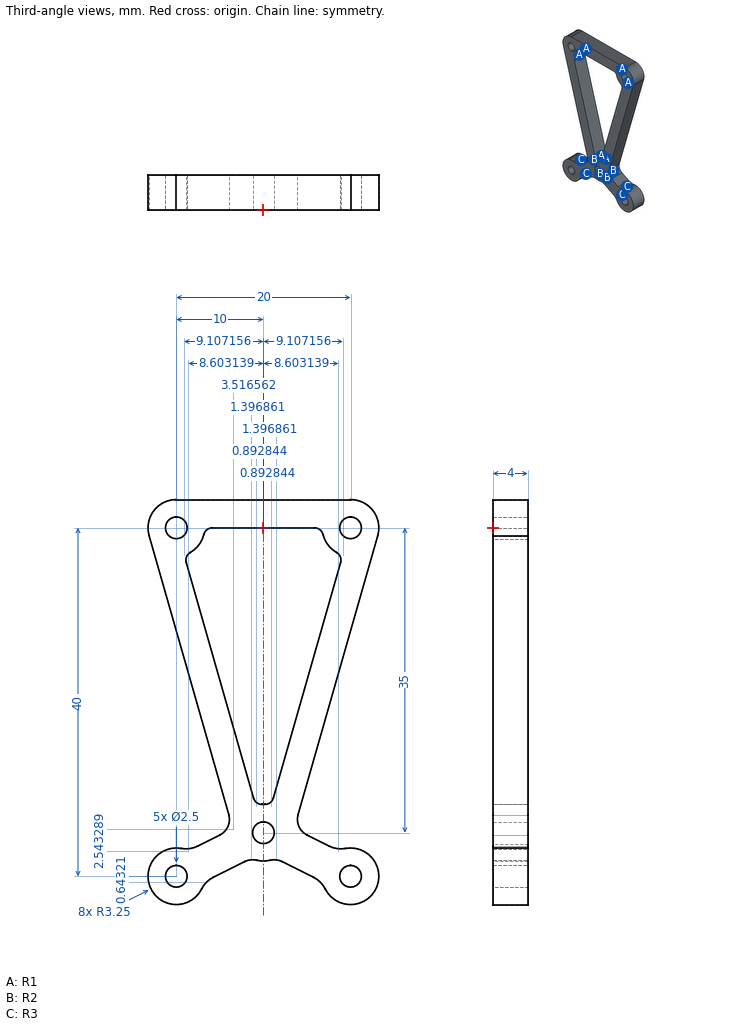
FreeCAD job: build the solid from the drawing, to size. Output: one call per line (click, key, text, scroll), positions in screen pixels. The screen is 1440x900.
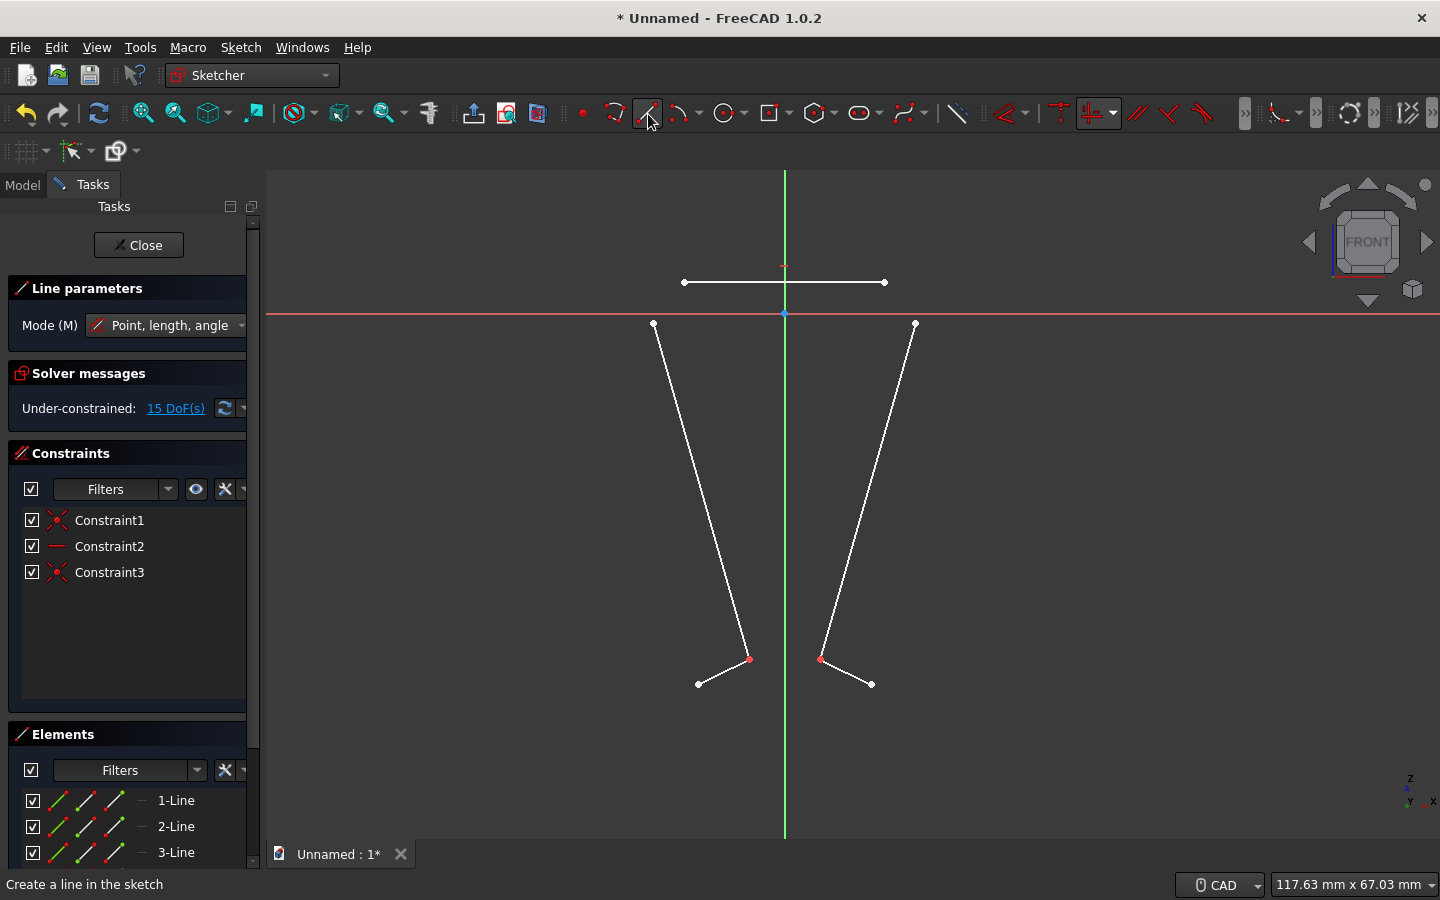
click(853, 720)
click(799, 693)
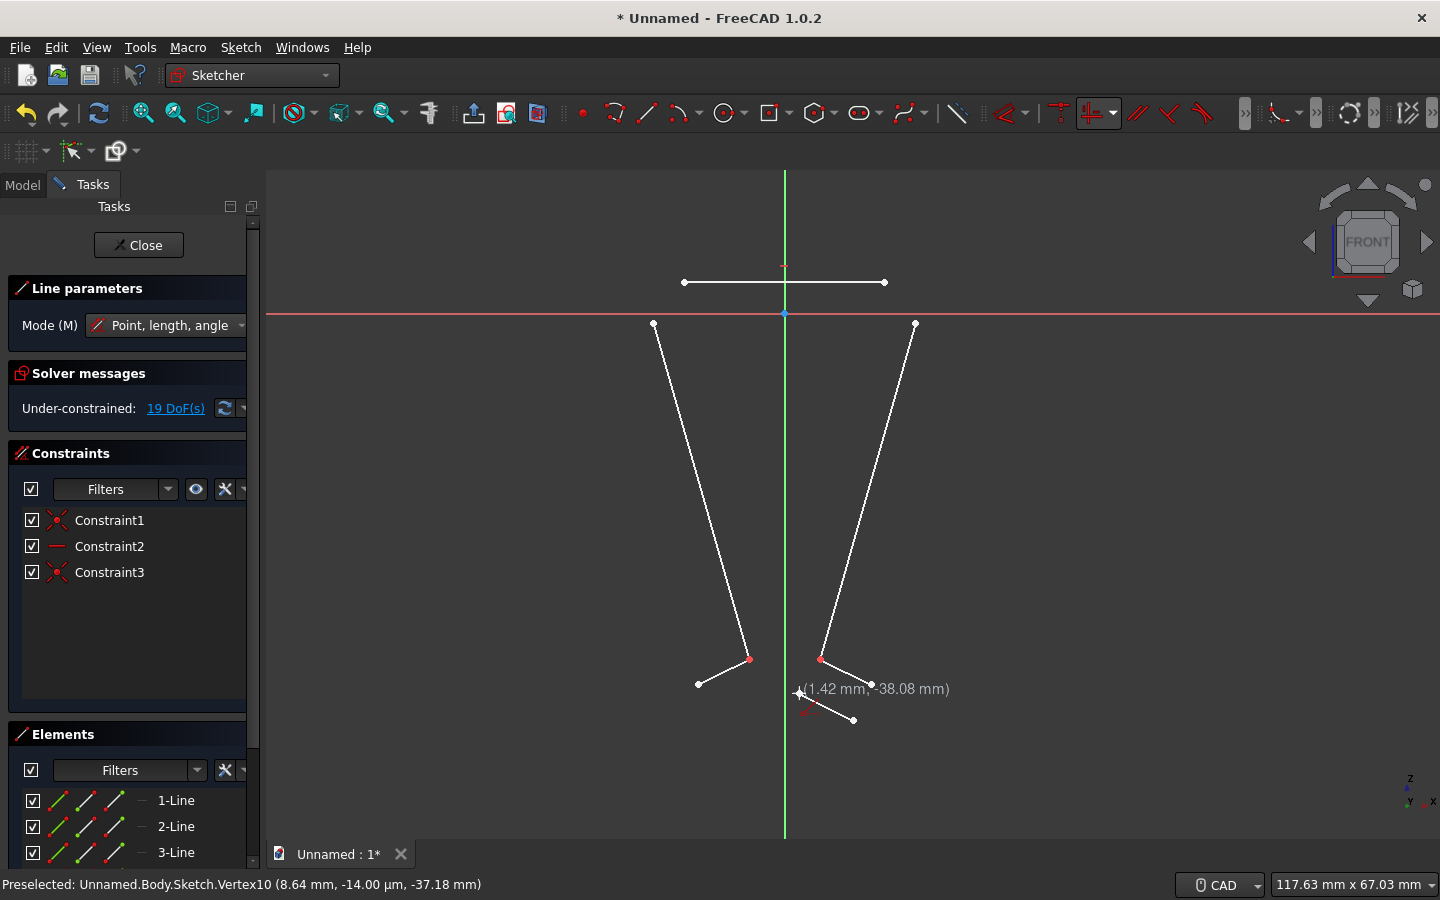
click(771, 693)
click(717, 720)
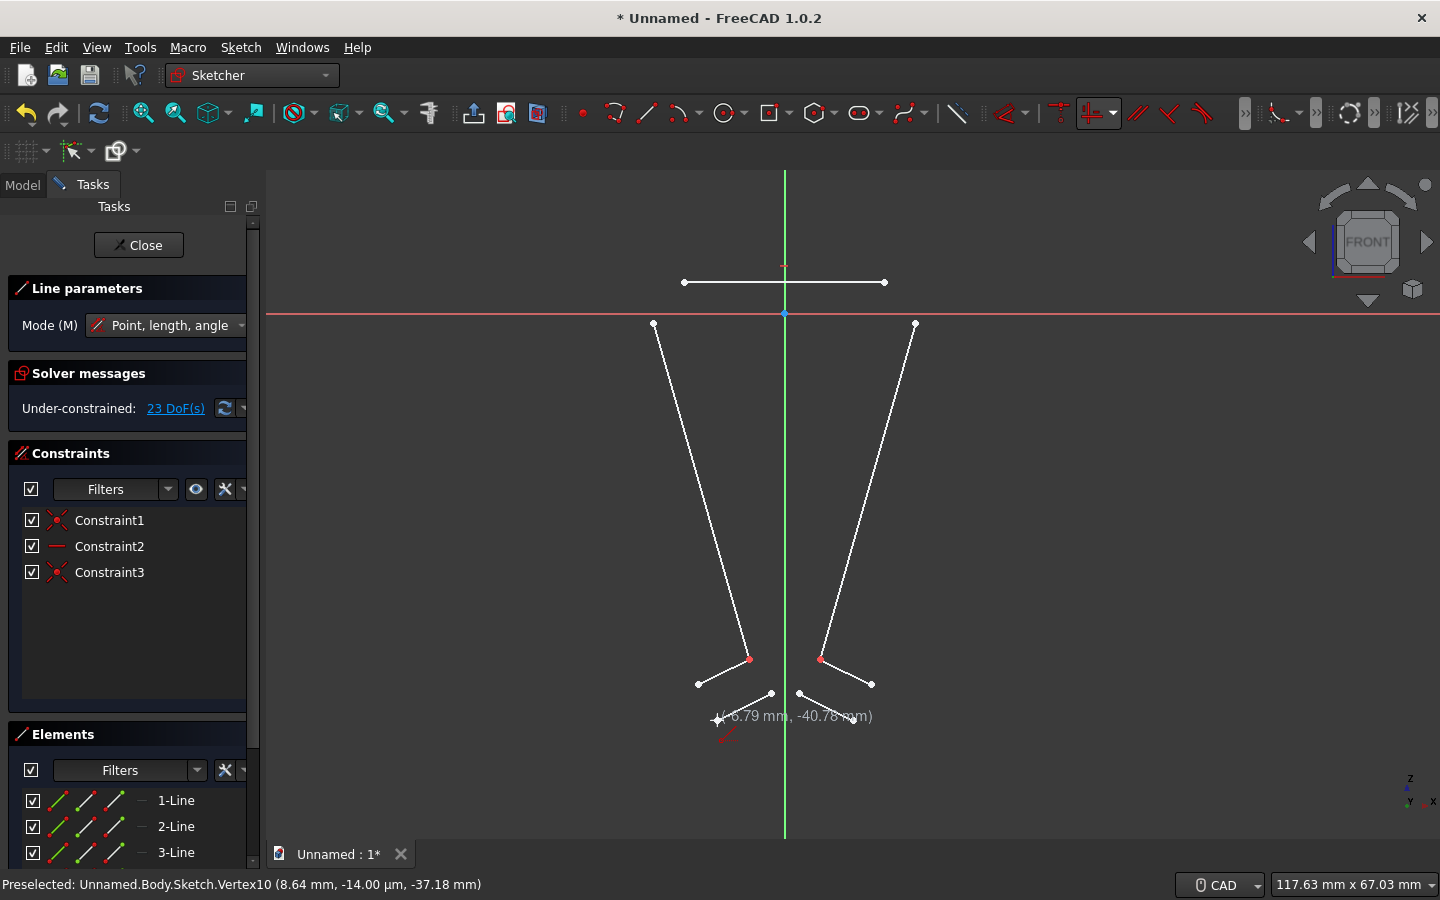
key(g)
key(3)
key(a)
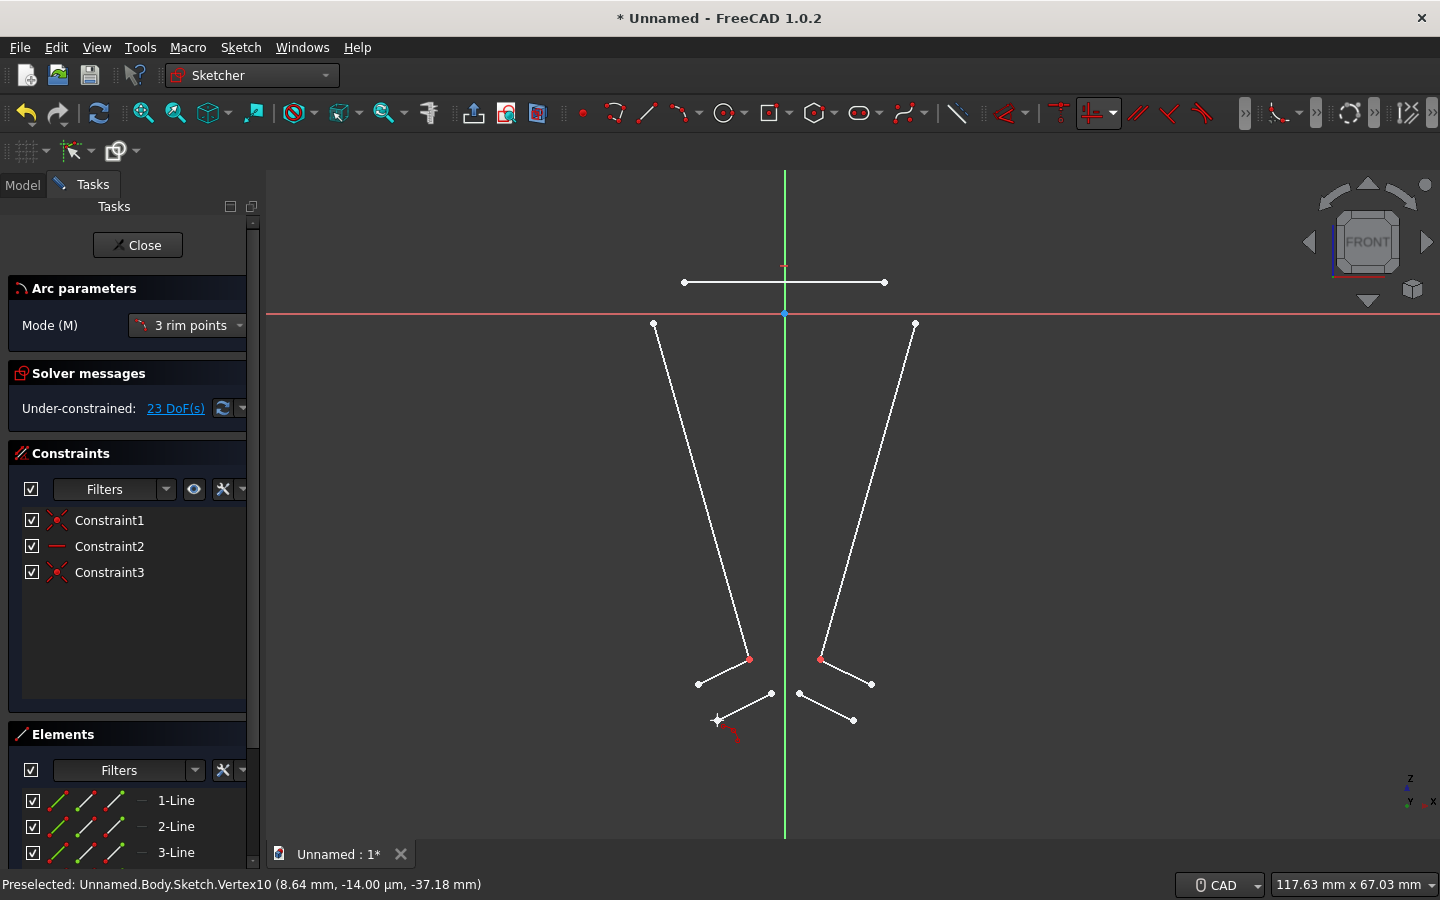
scroll(654, 323, up, 3)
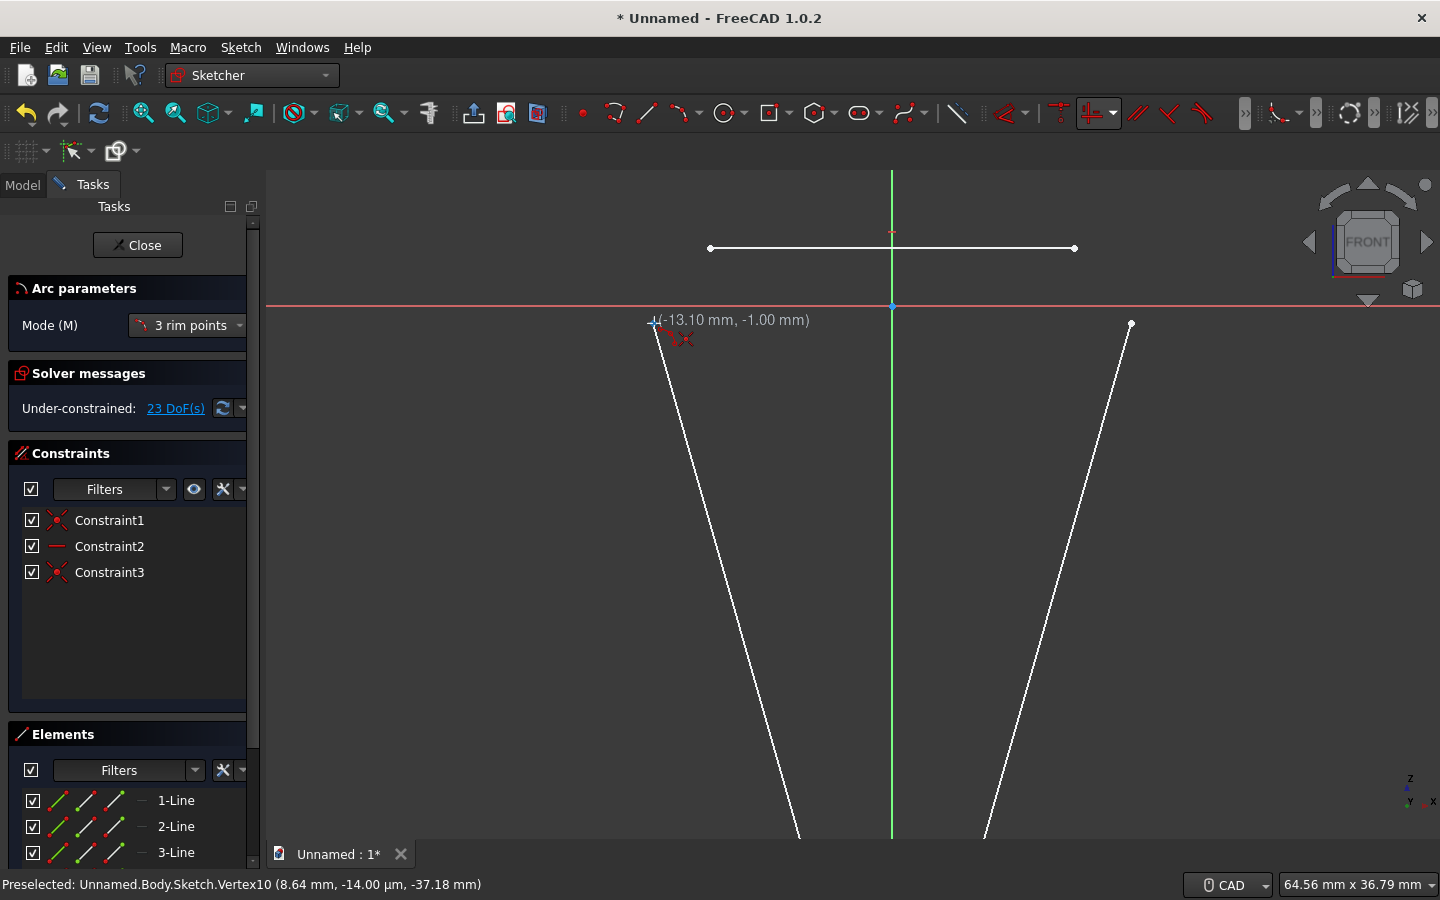
click(653, 323)
click(710, 248)
click(663, 271)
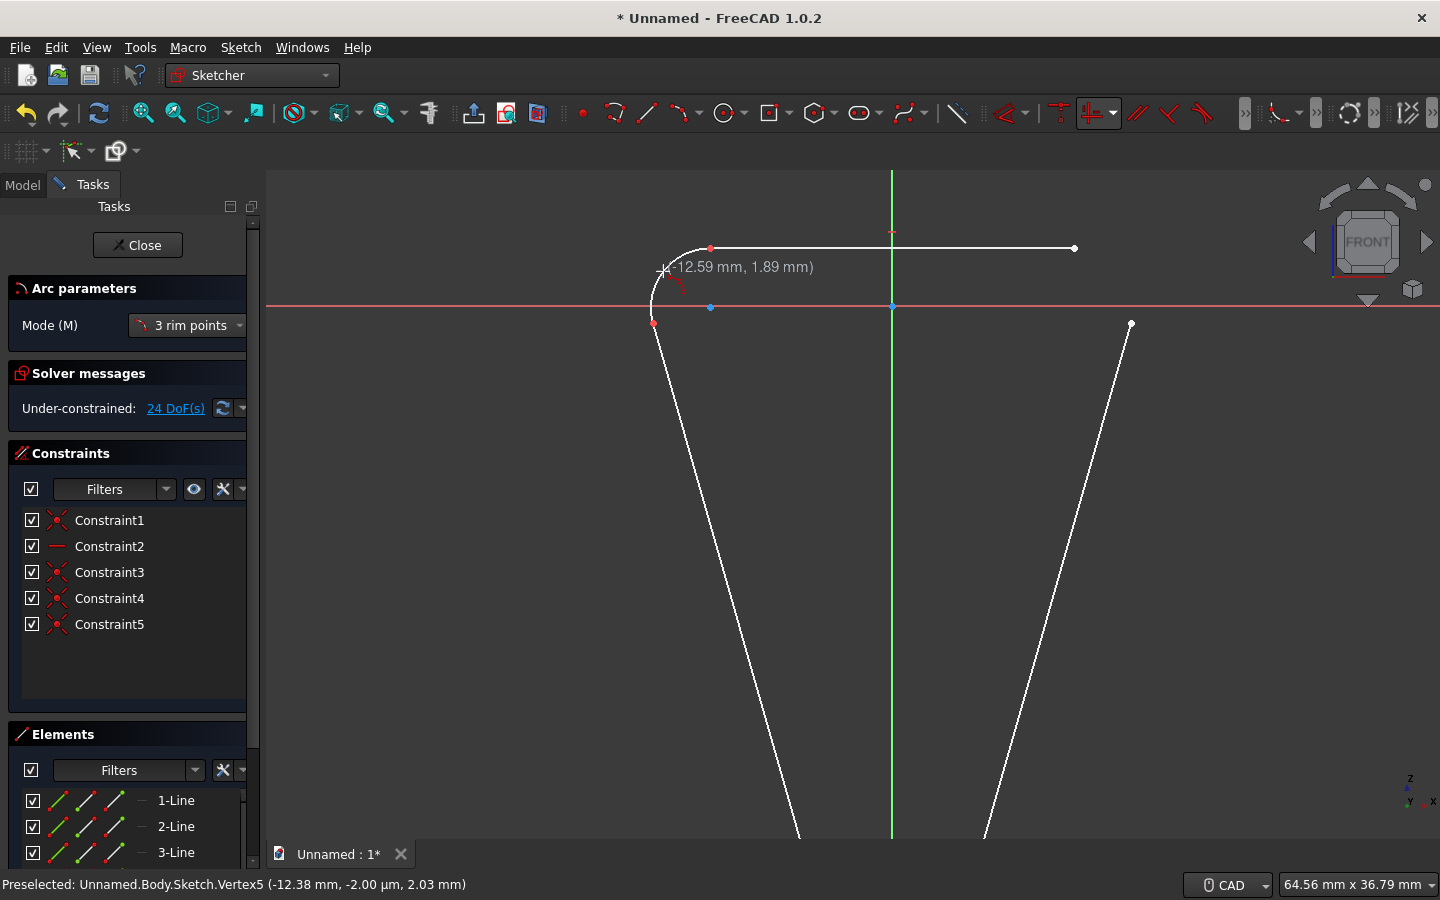
click(1074, 248)
click(1131, 323)
click(1121, 271)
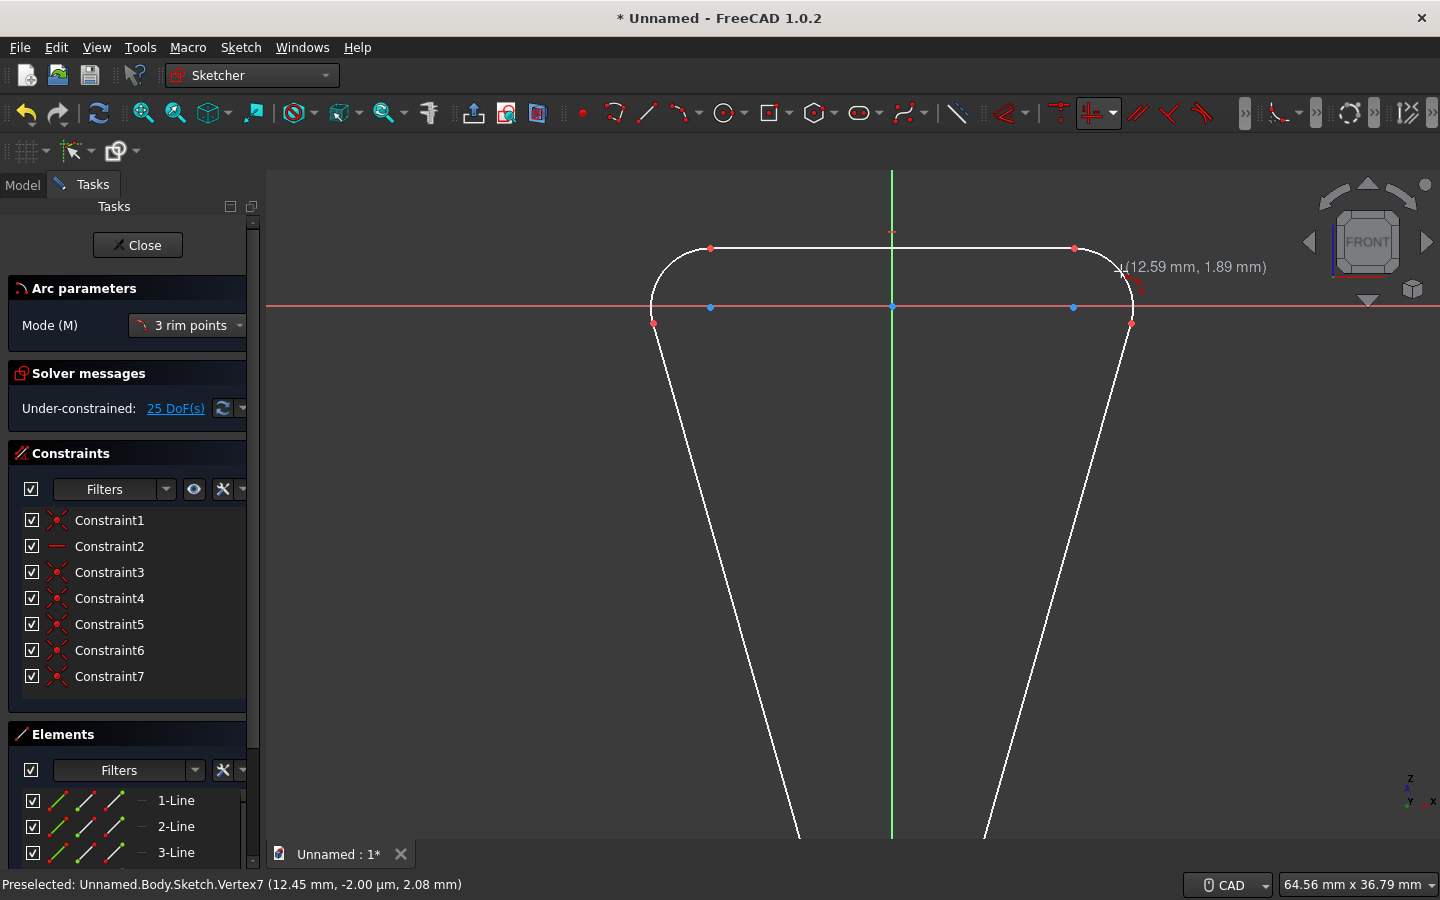
scroll(654, 323, down, 3)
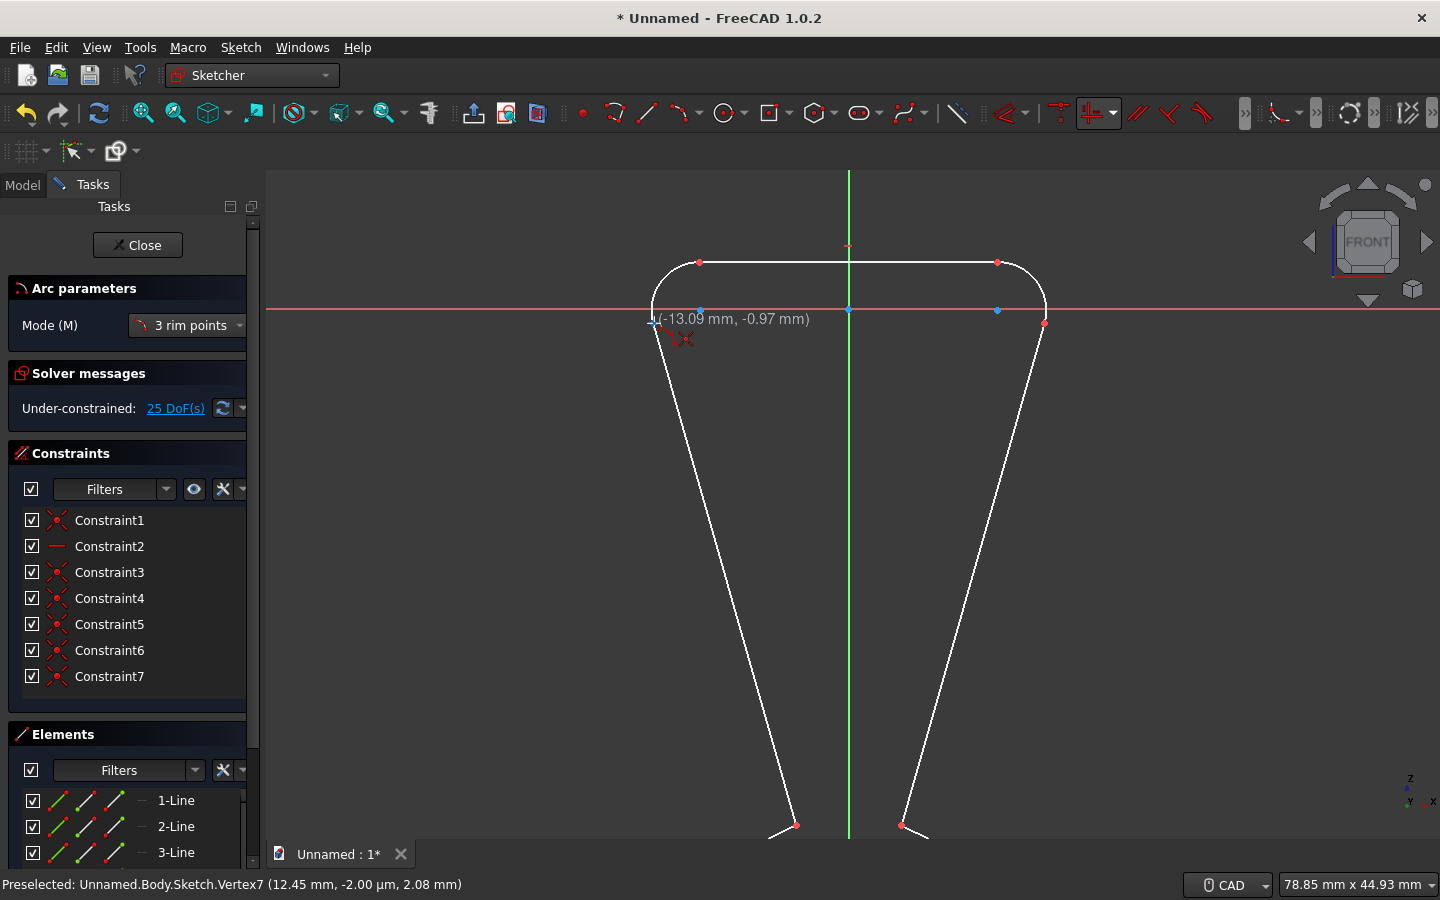
click(871, 685)
click(853, 721)
click(914, 728)